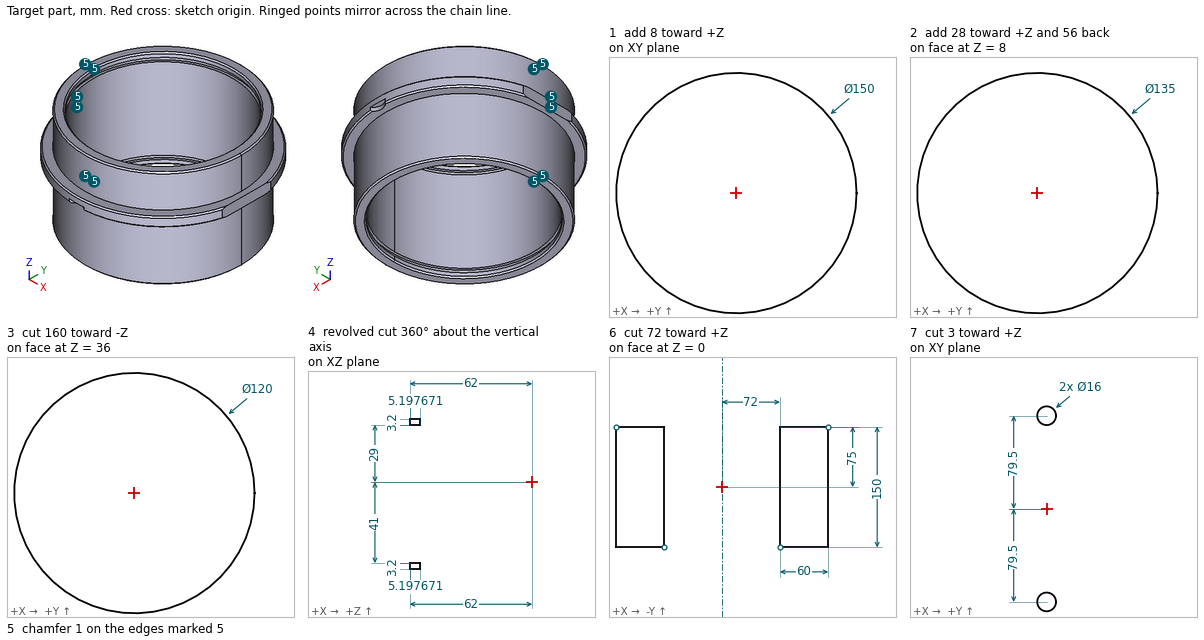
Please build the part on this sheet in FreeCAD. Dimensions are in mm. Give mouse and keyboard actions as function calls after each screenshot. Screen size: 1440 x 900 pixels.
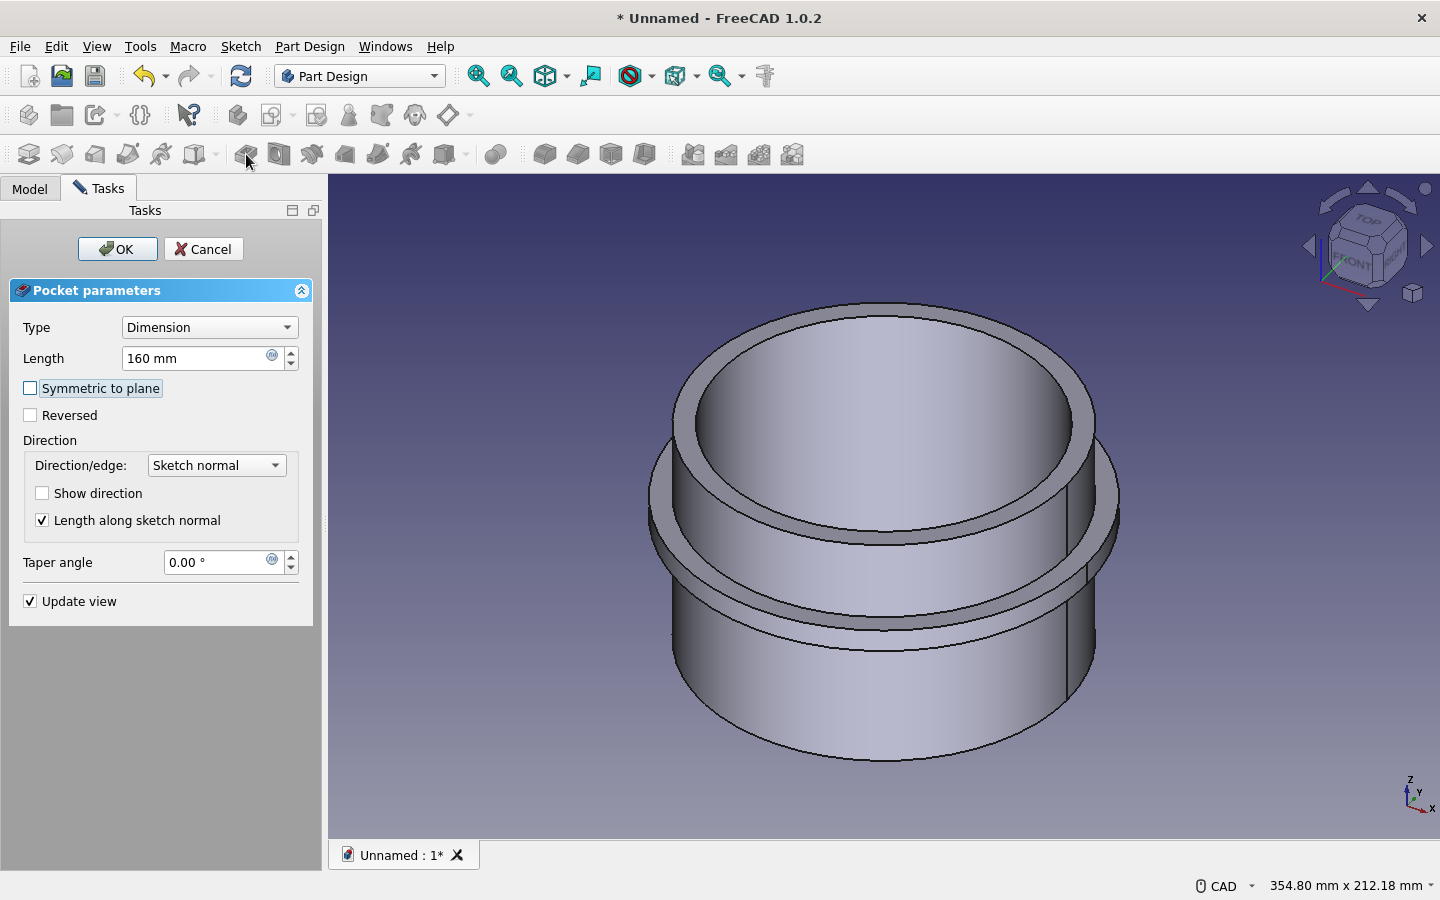
click(118, 249)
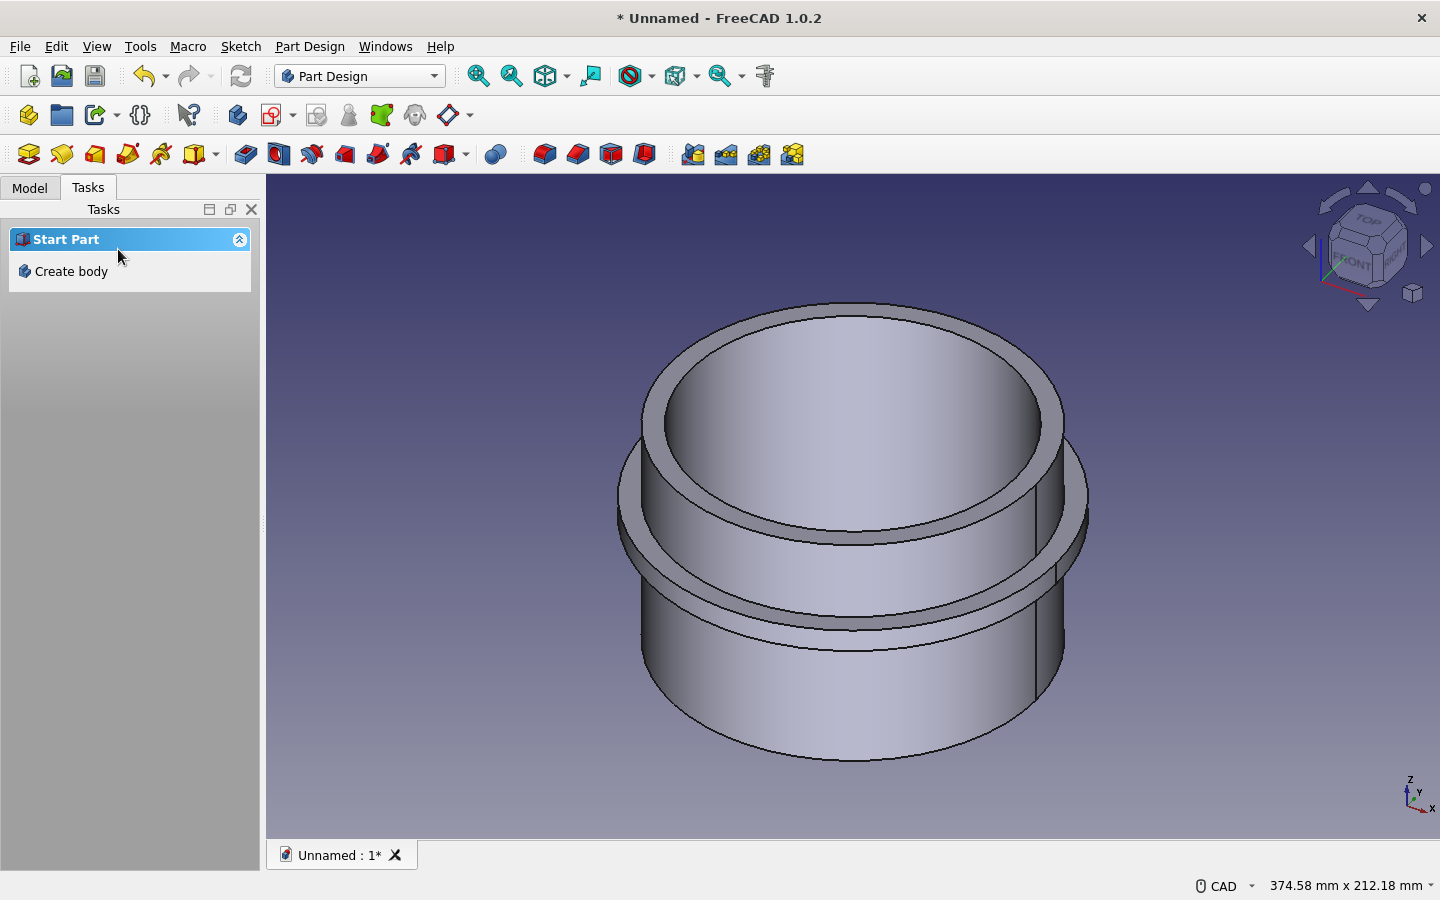
click(270, 116)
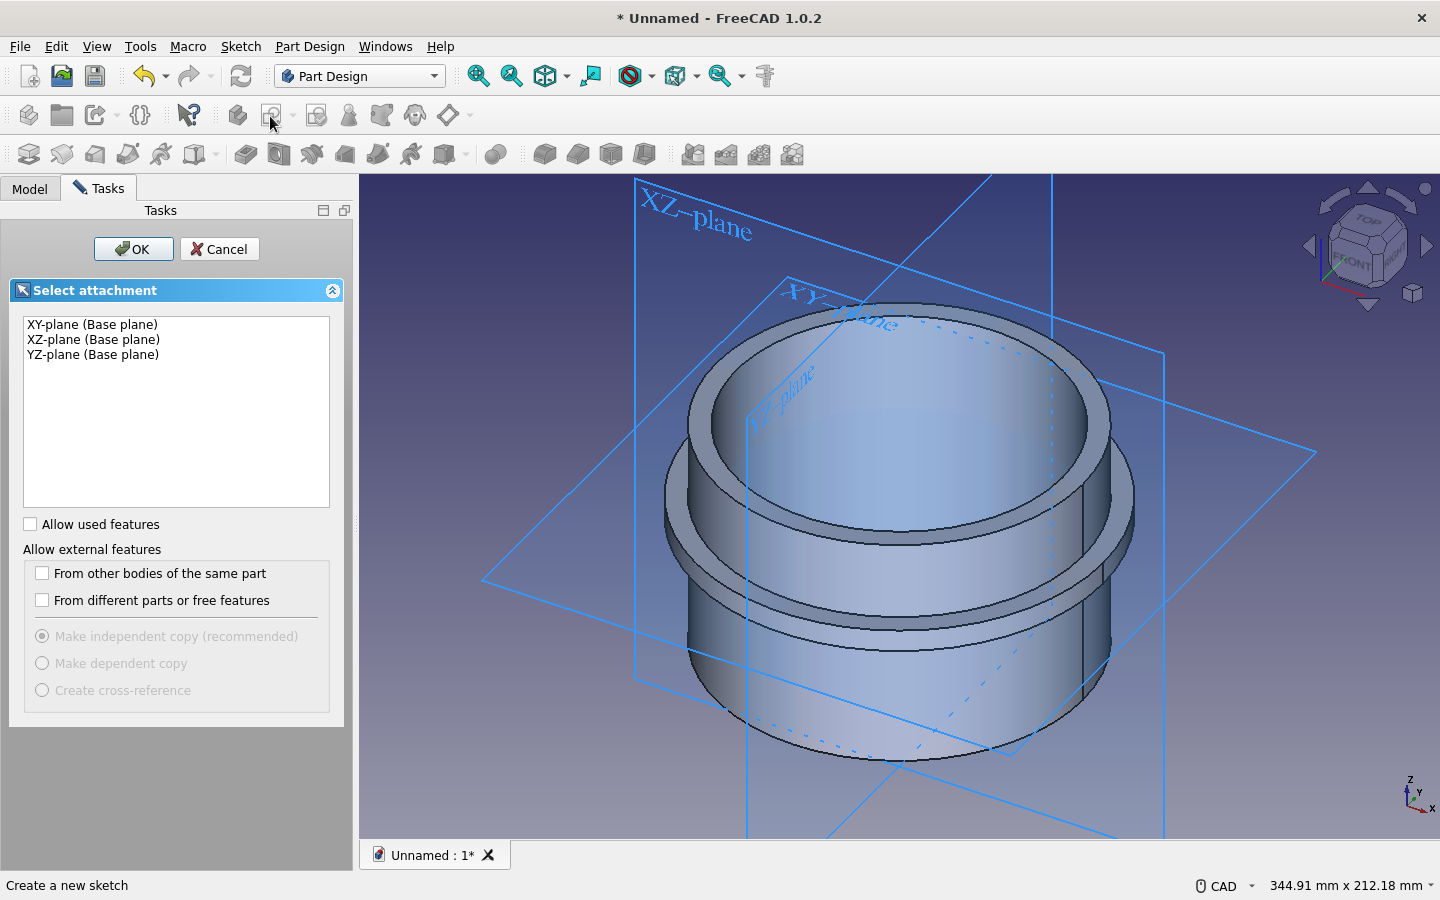
click(84, 340)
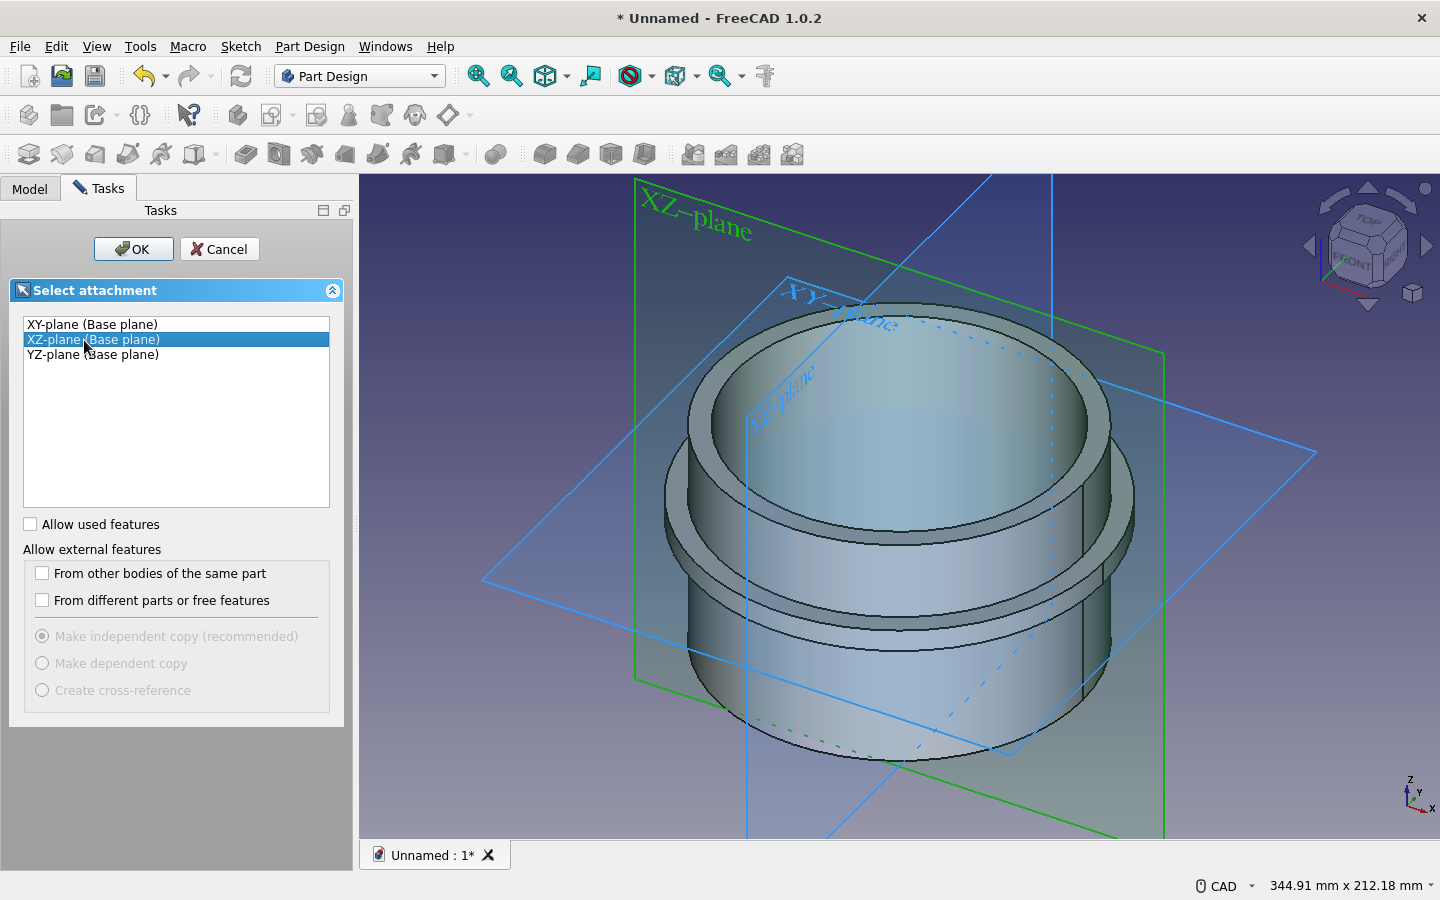
click(134, 249)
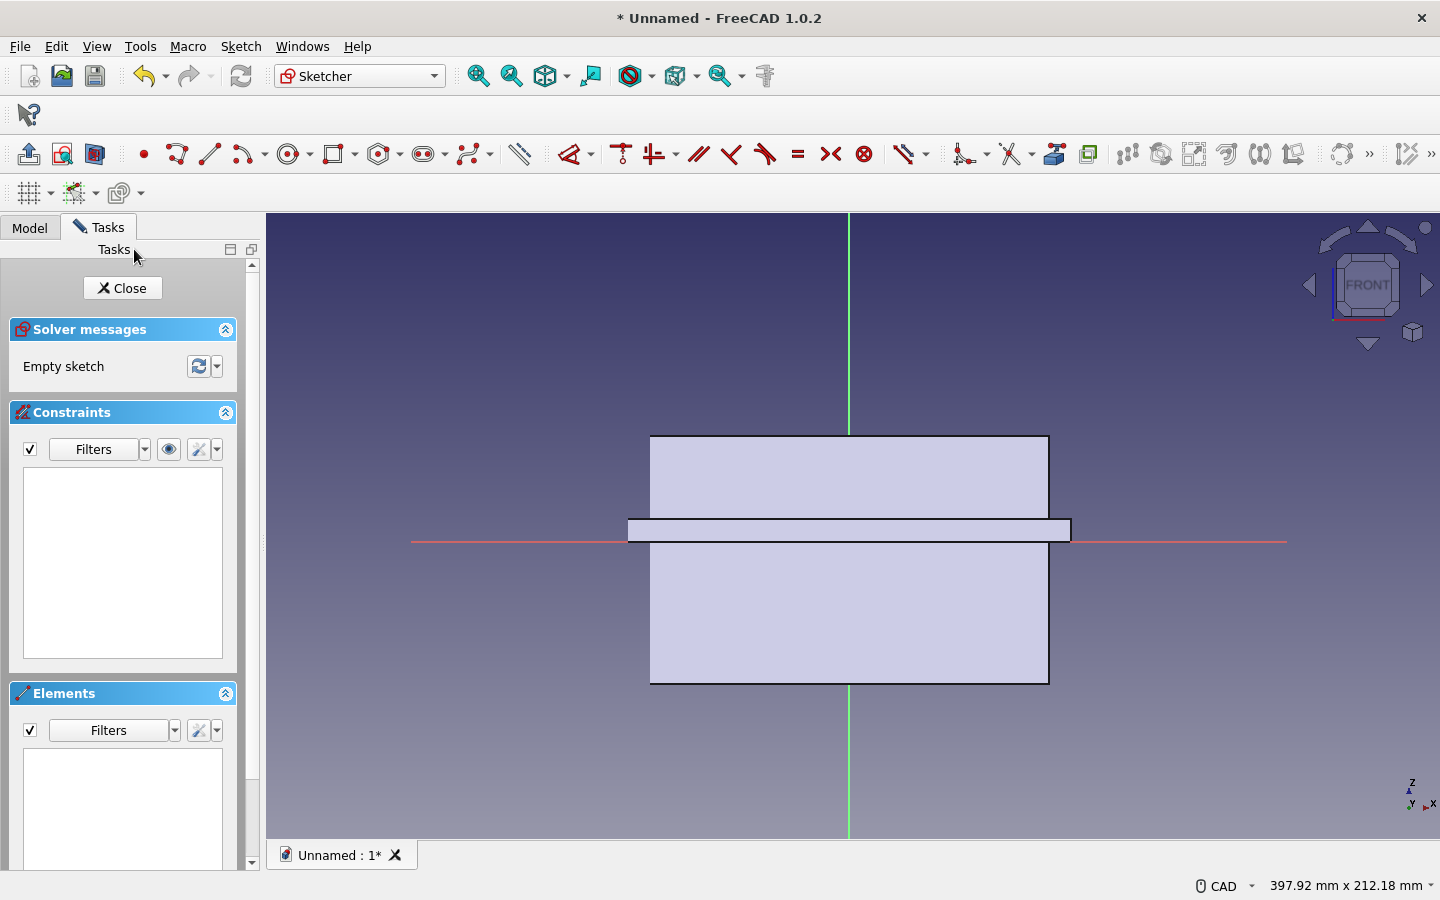
key(q)
key(s)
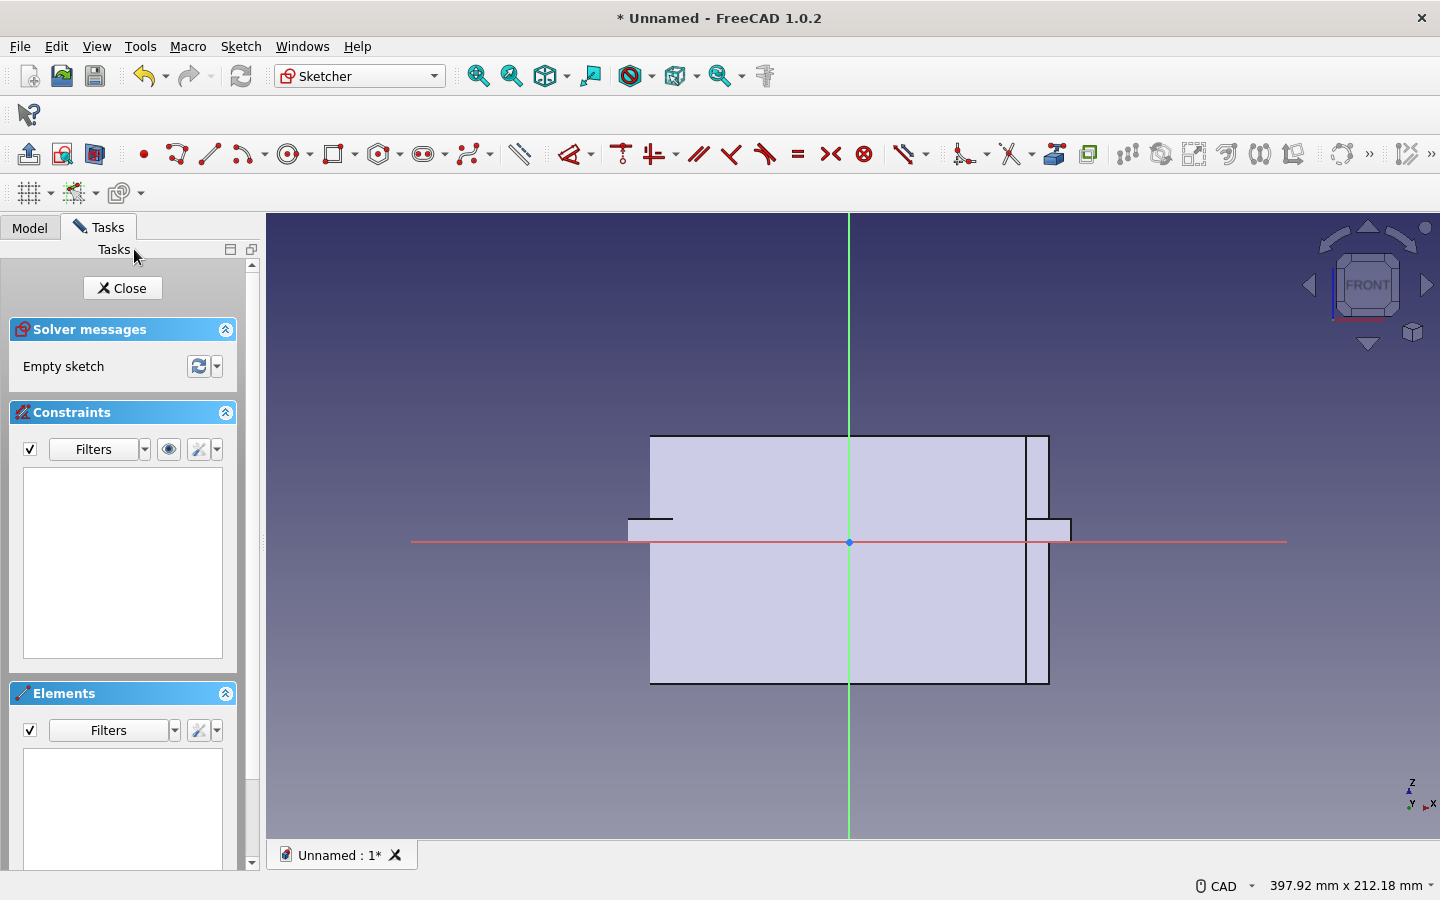
scroll(726, 601, up, 3)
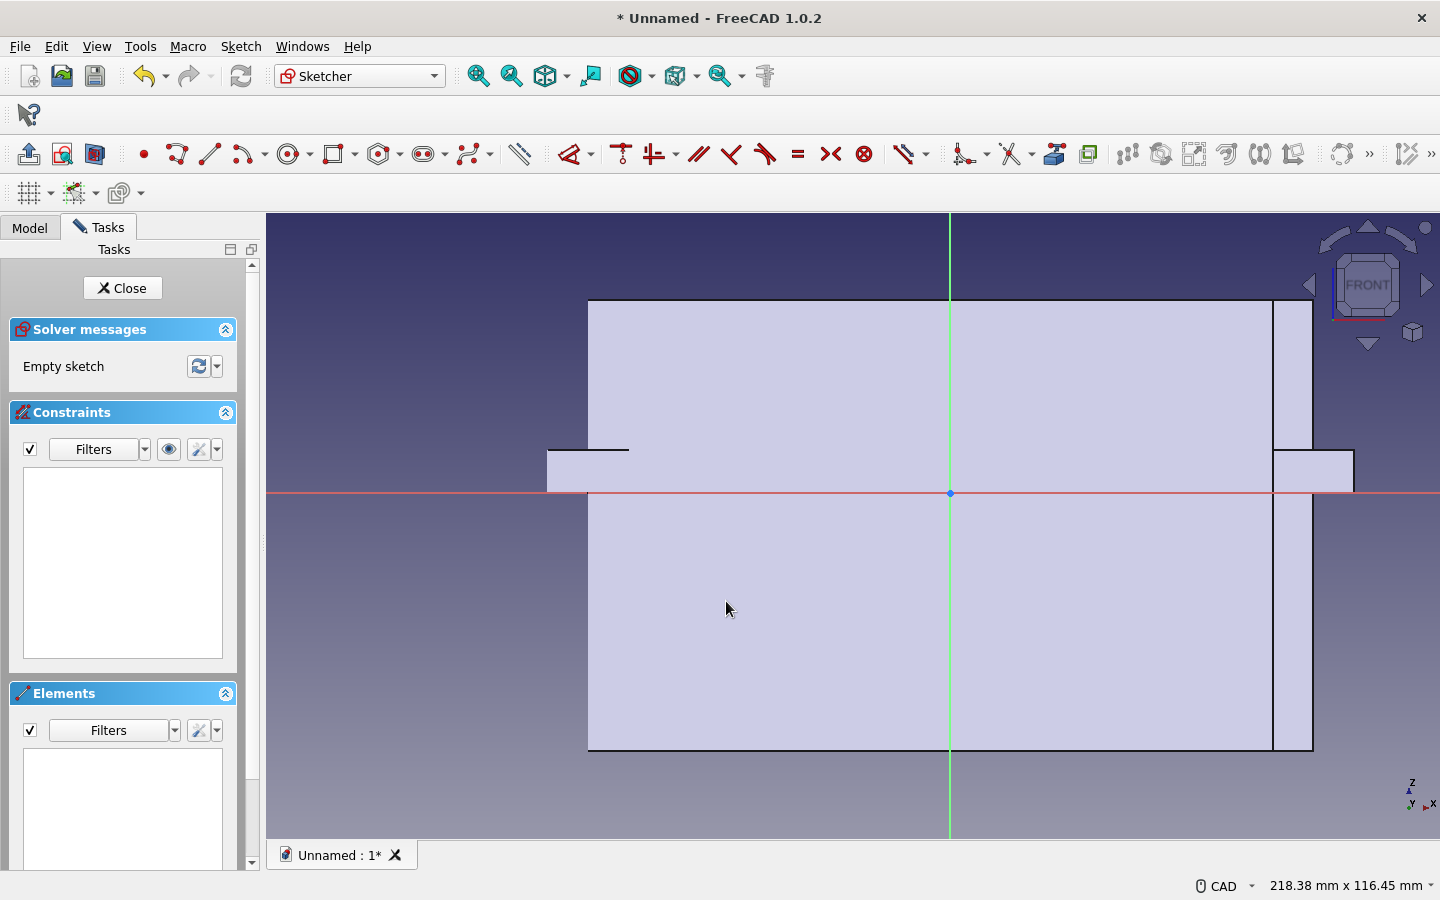
click(332, 154)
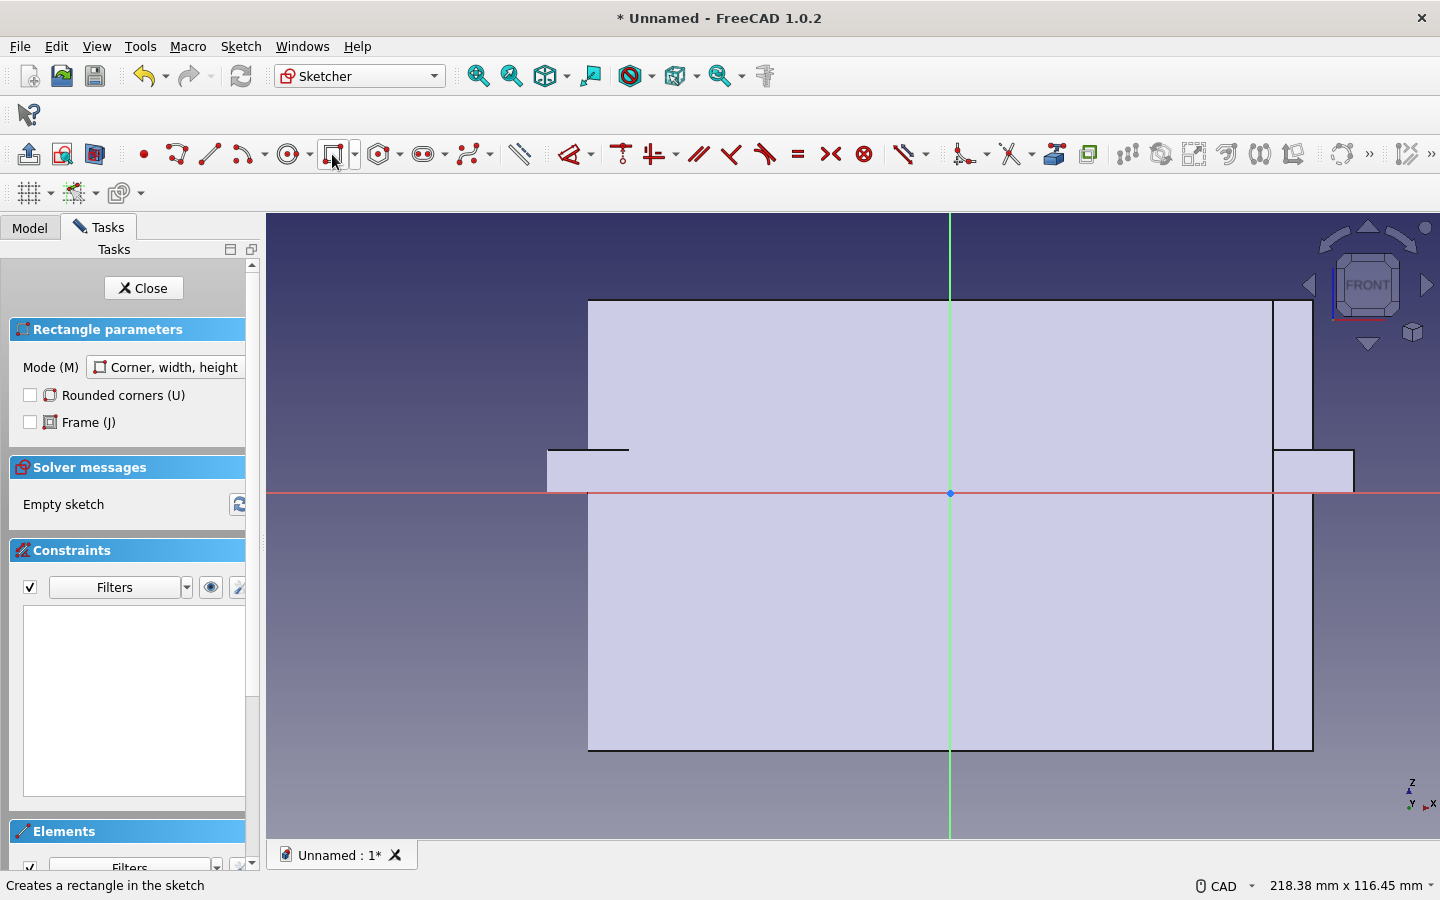
click(617, 320)
click(645, 337)